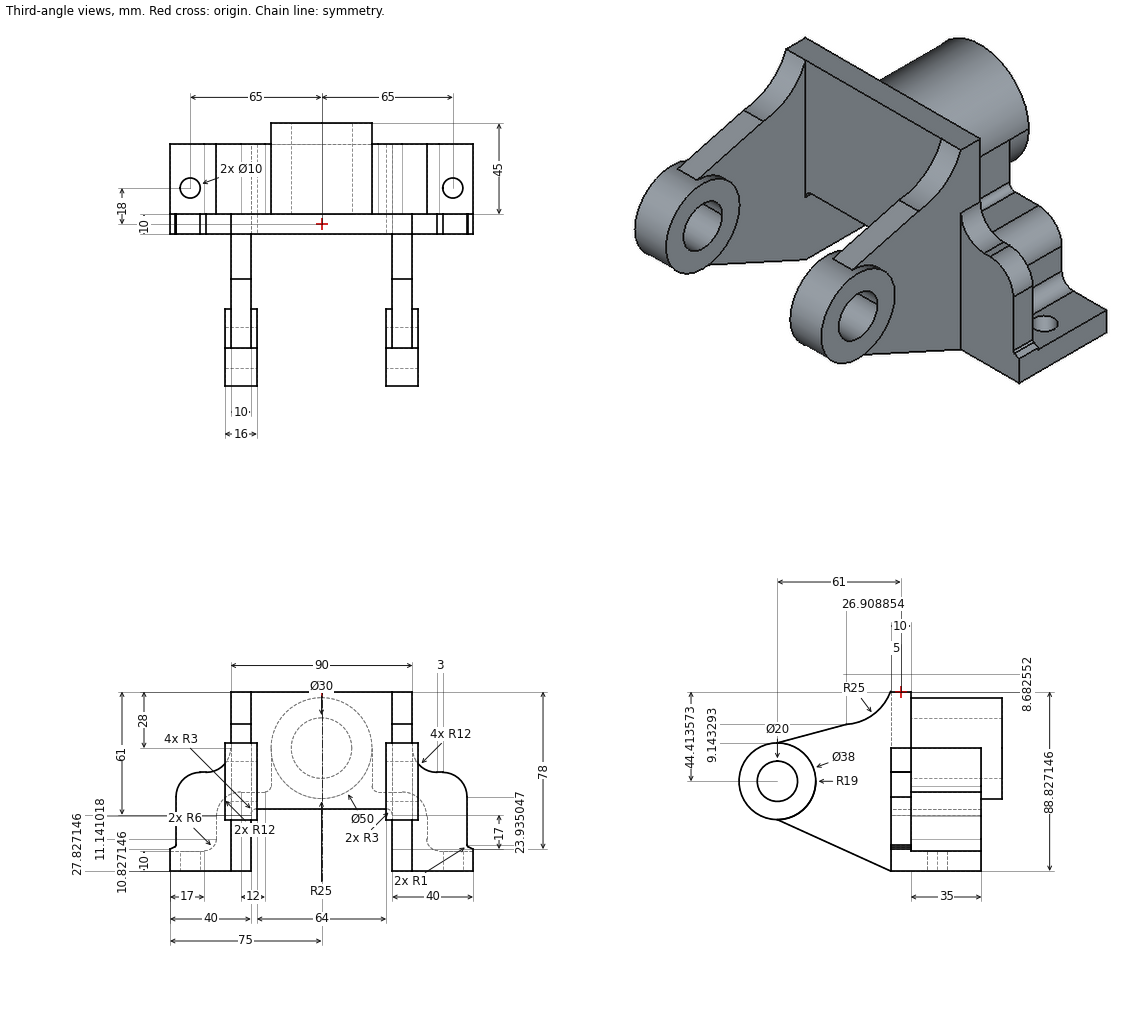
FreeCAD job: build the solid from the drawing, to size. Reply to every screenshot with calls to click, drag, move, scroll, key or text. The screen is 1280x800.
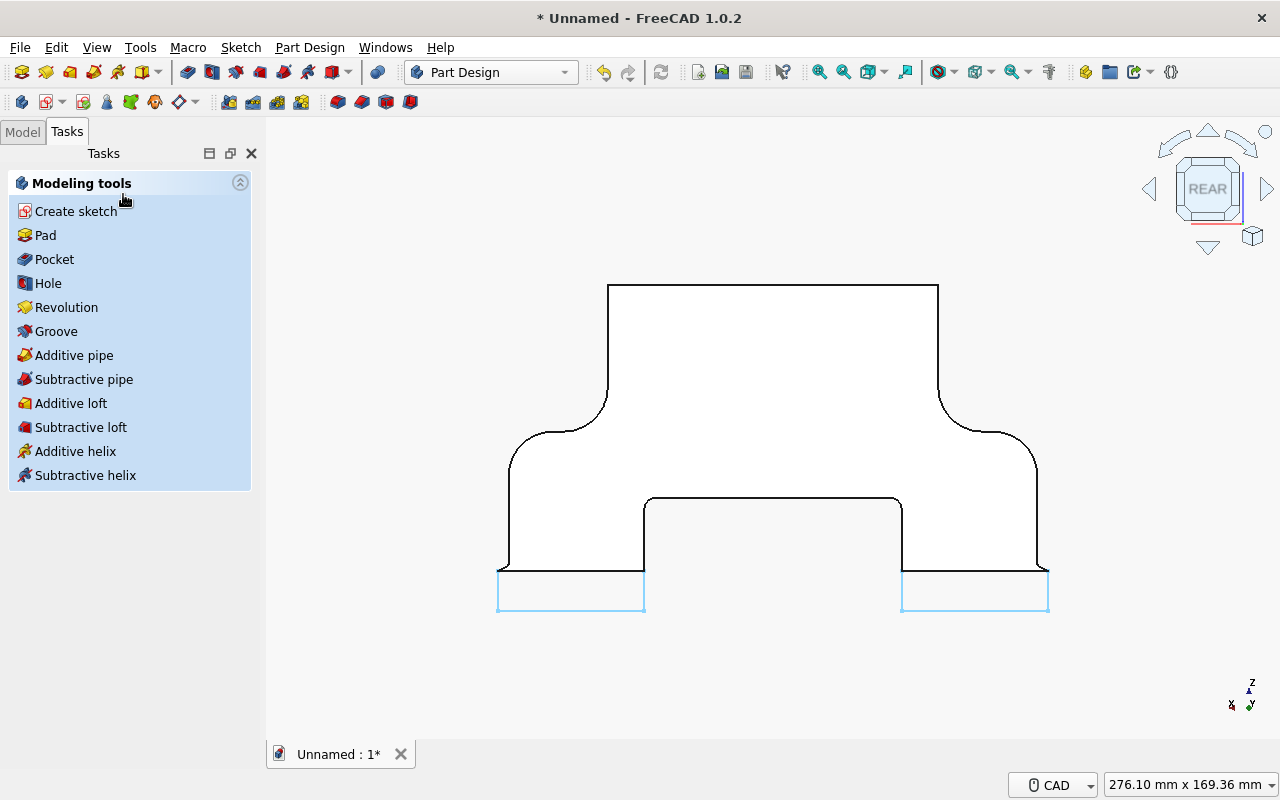
click(22, 72)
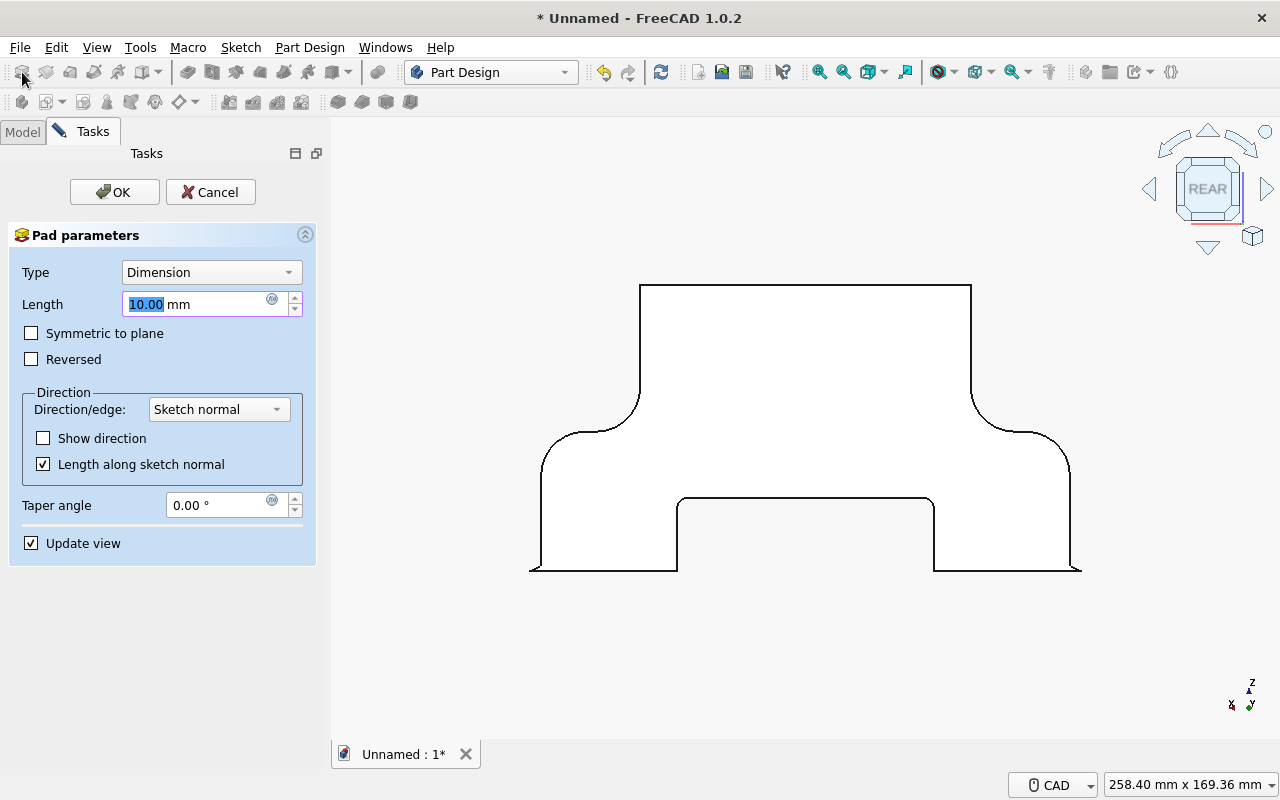
text(10)
key(Tab)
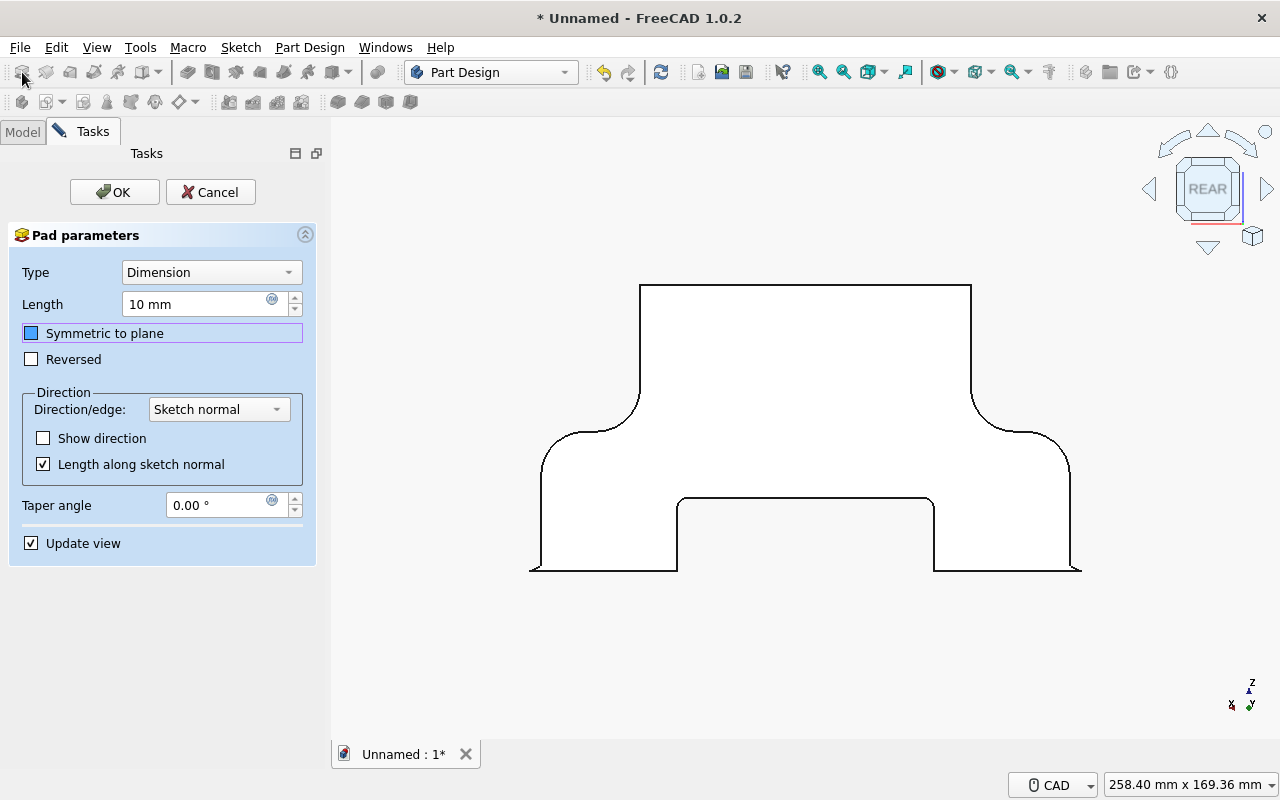
click(30, 359)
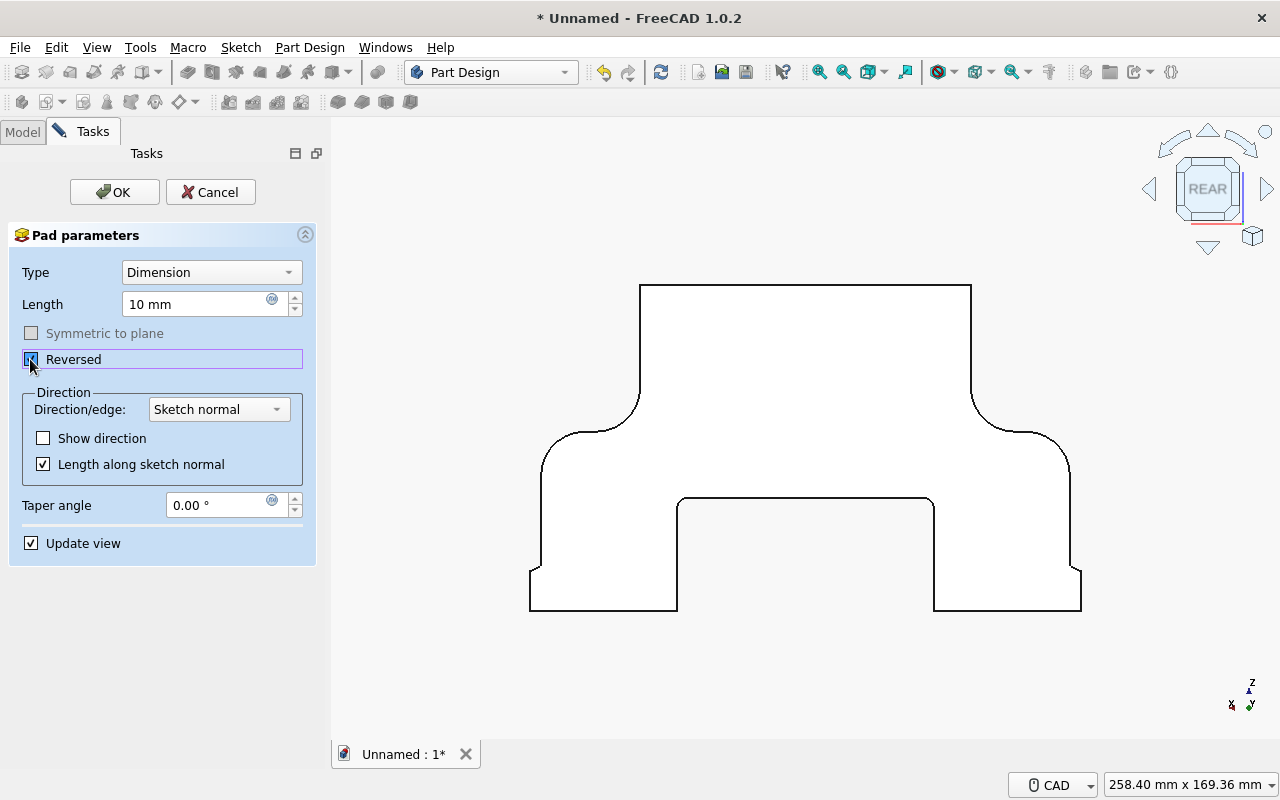
click(115, 192)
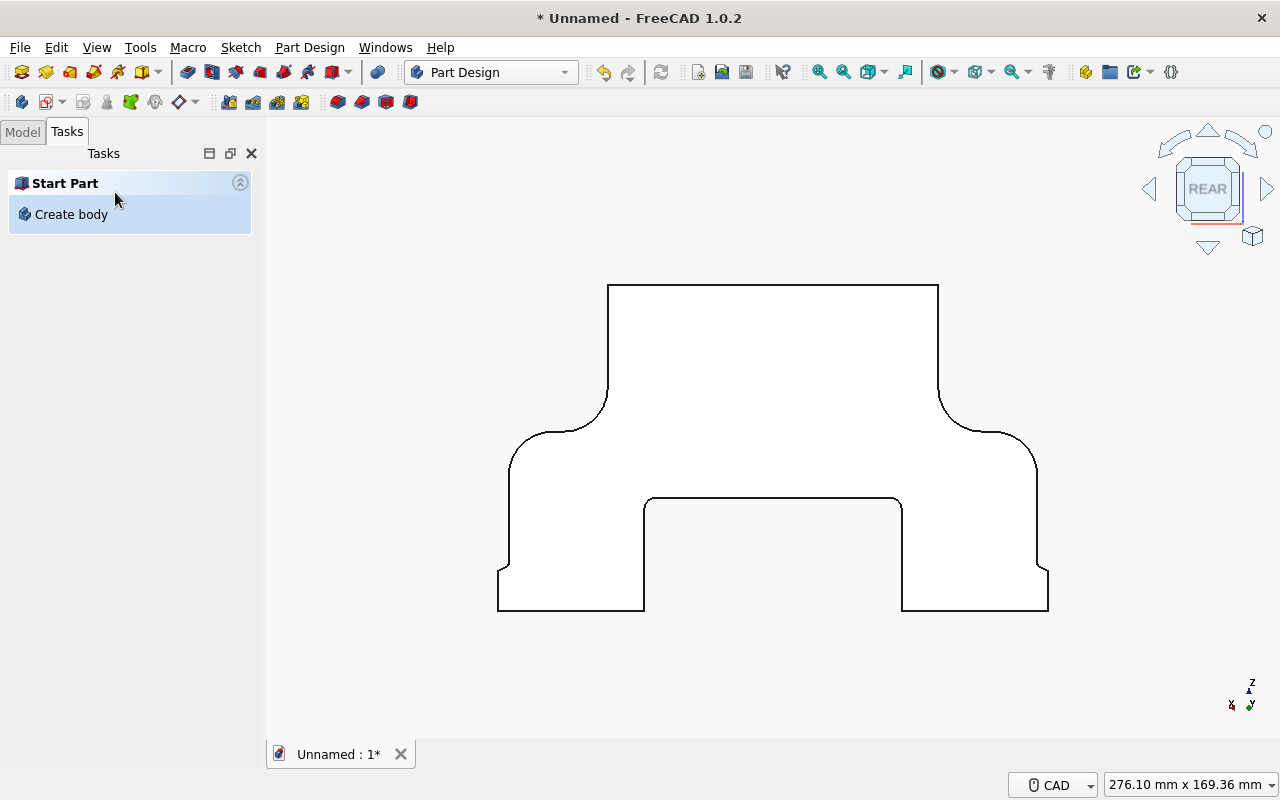
click(23, 131)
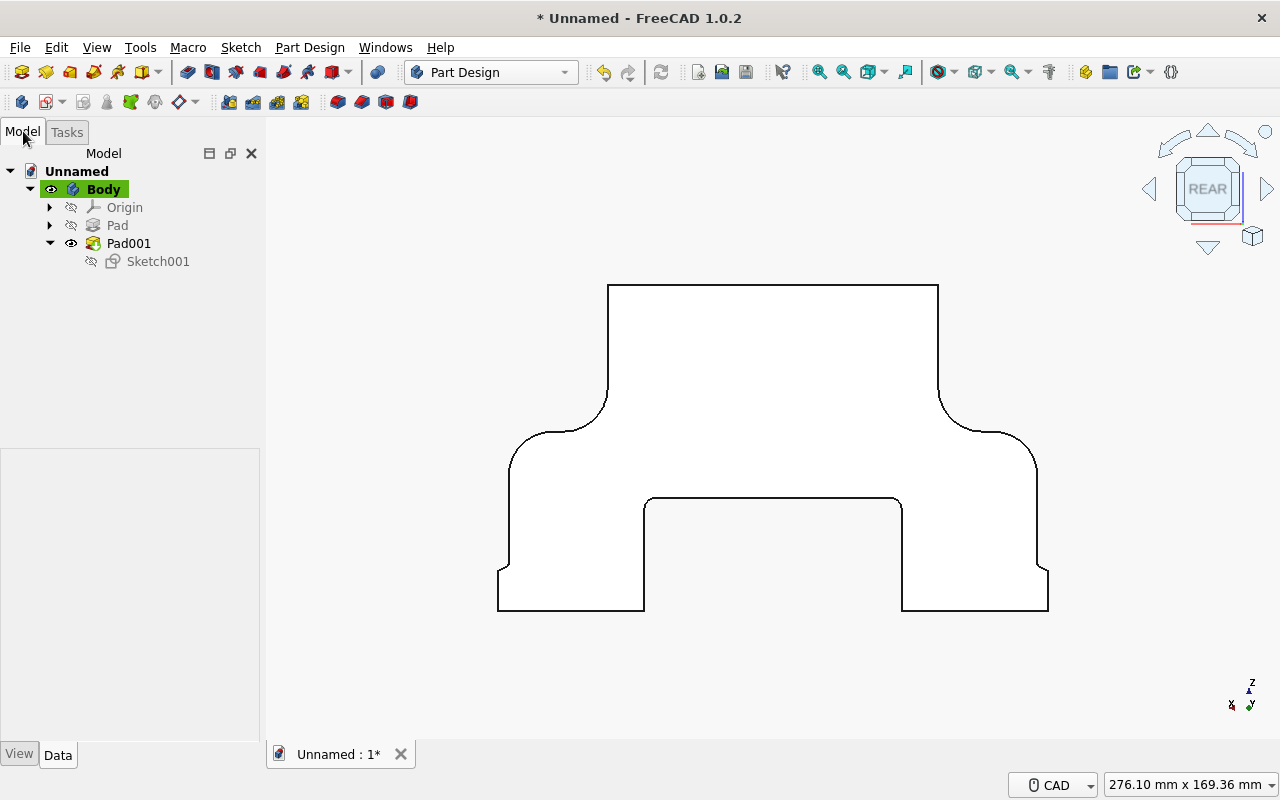
click(50, 207)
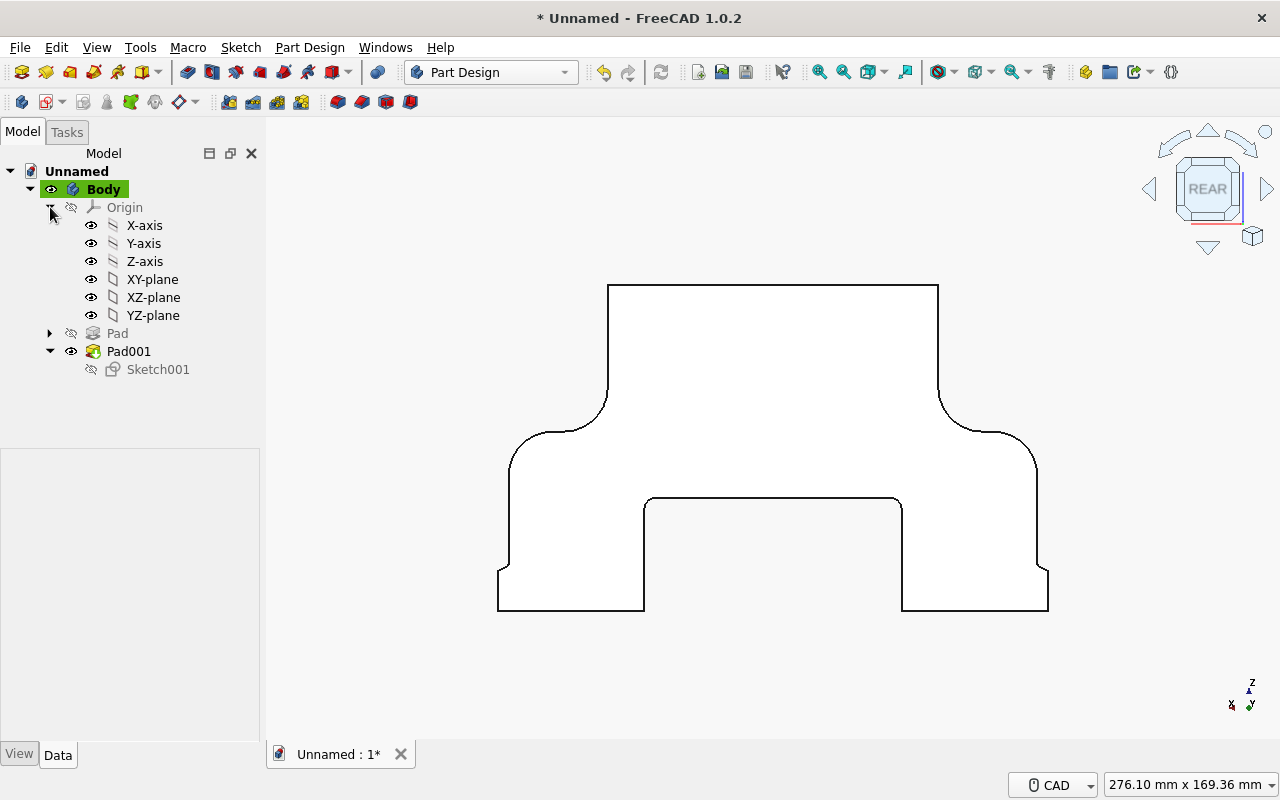
click(136, 297)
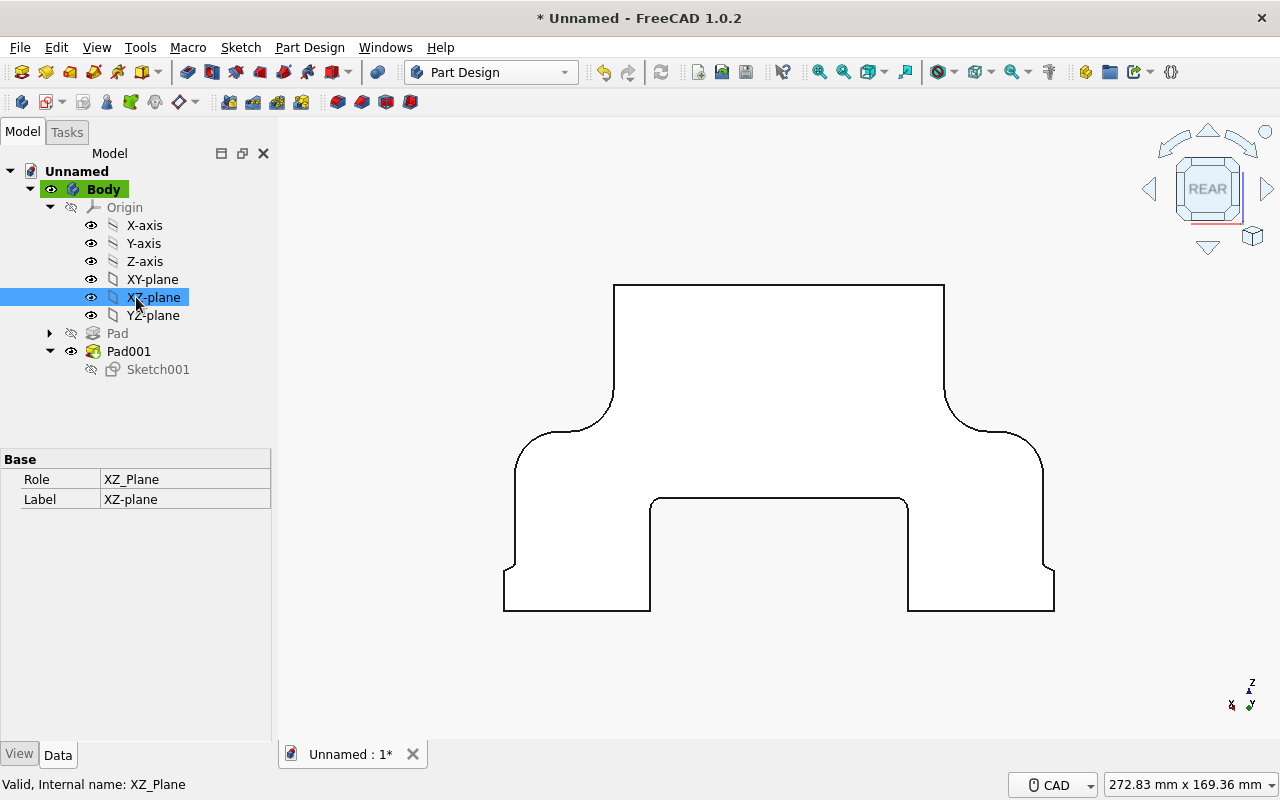
click(180, 102)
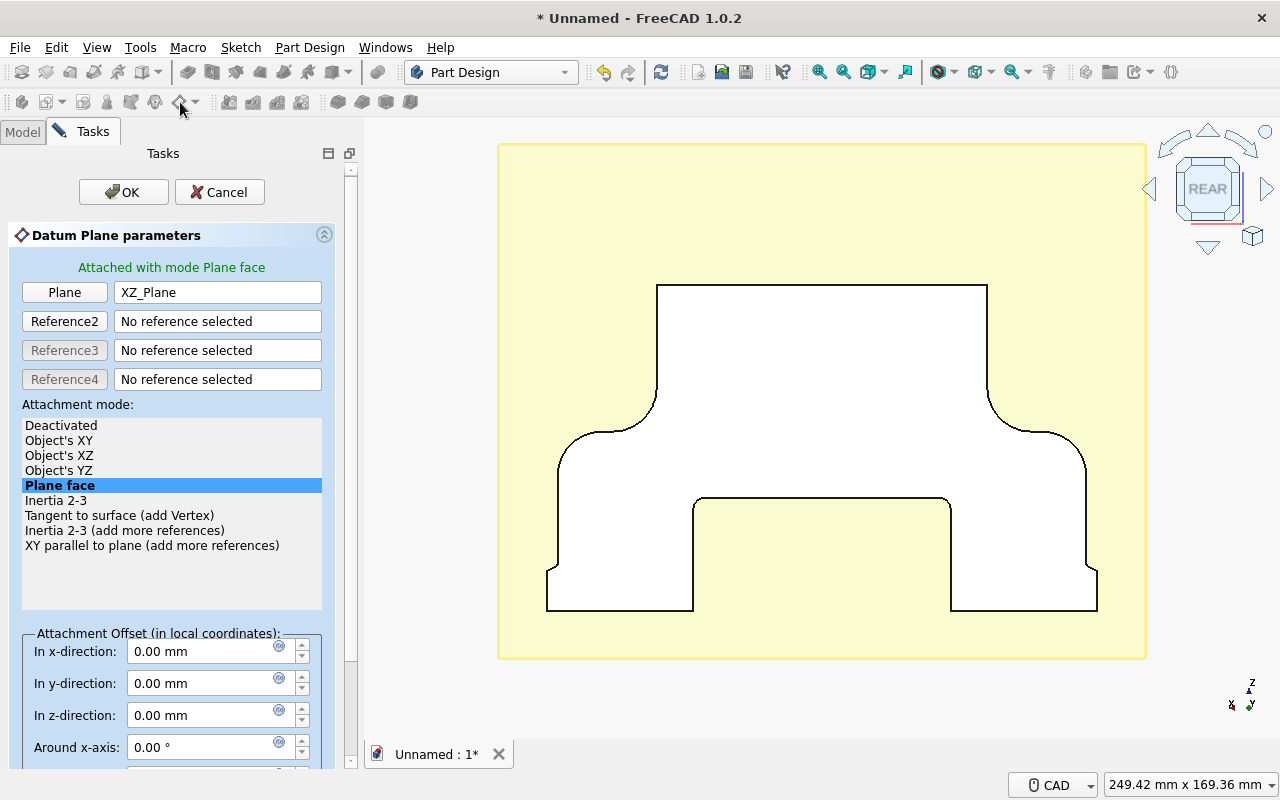
triple_click(210, 715)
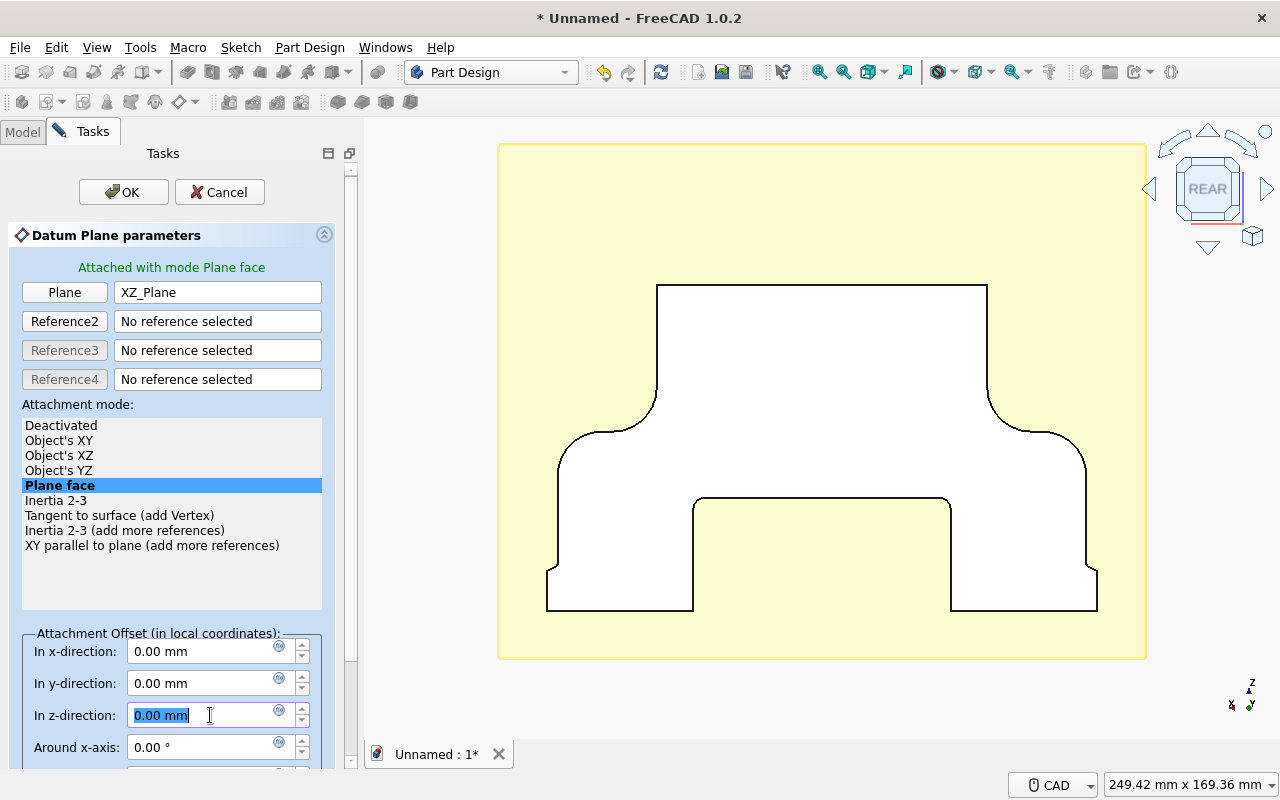
text(-40)
key(Tab)